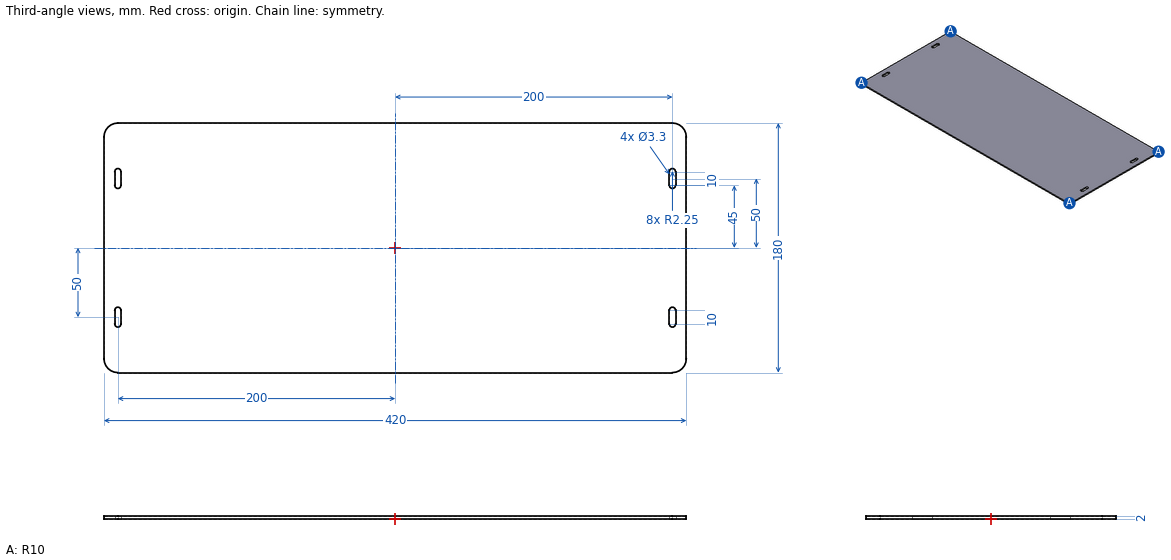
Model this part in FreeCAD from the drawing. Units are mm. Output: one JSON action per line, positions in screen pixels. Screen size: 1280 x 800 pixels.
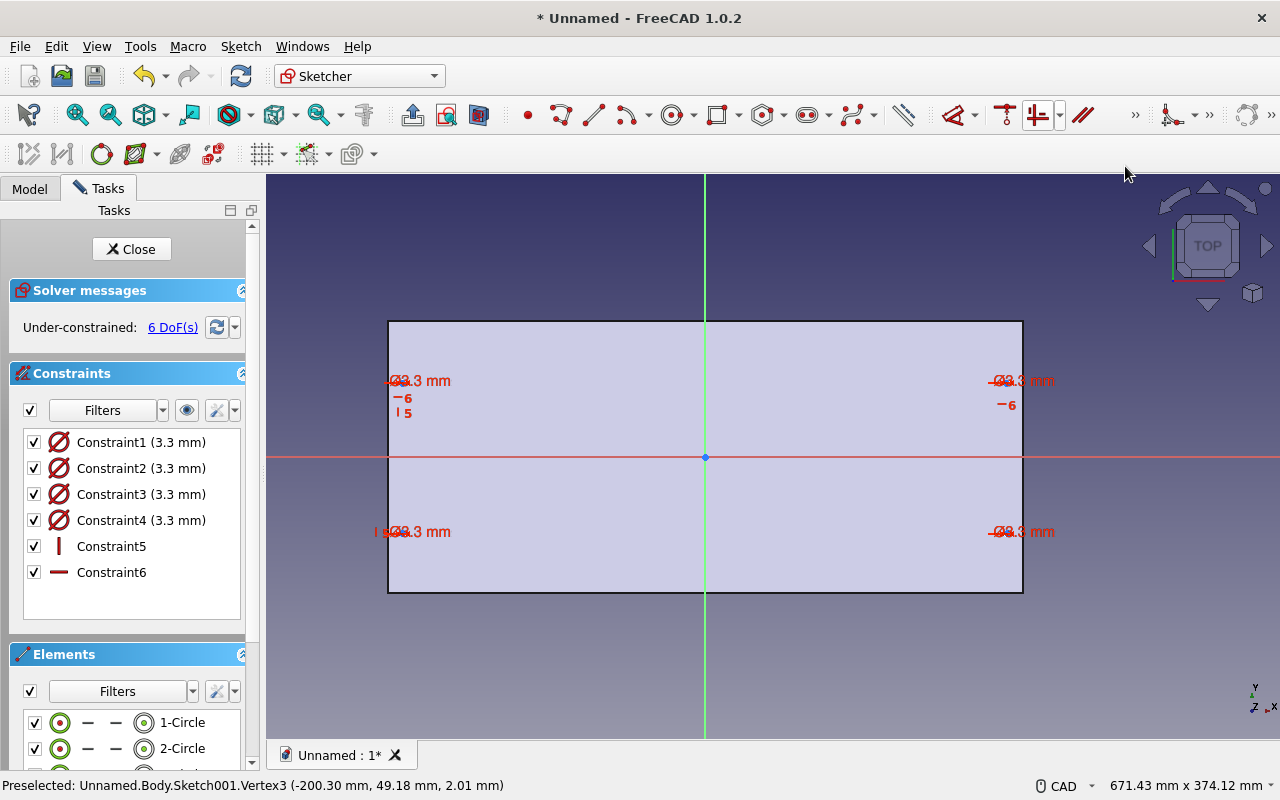
{"action": "left_click", "coordinate": [1007, 383]}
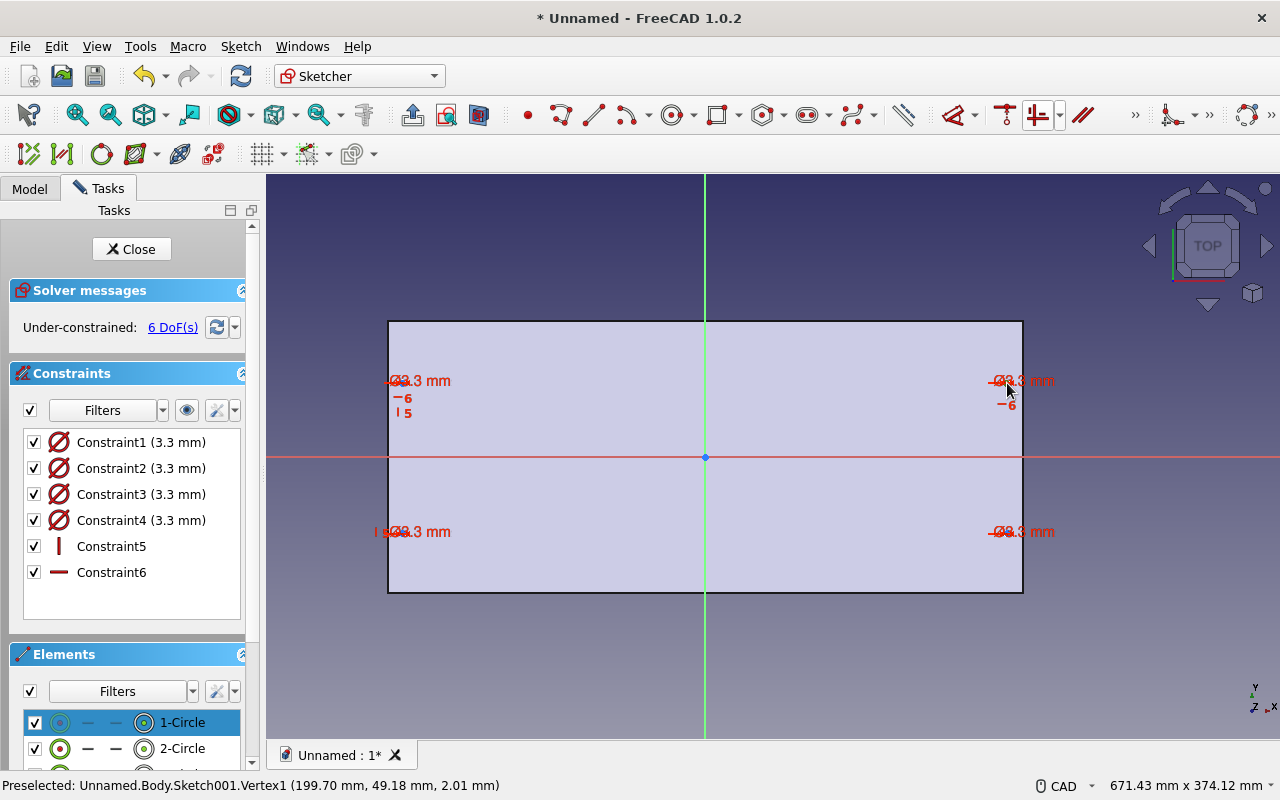
{"action": "left_click", "coordinate": [1007, 534]}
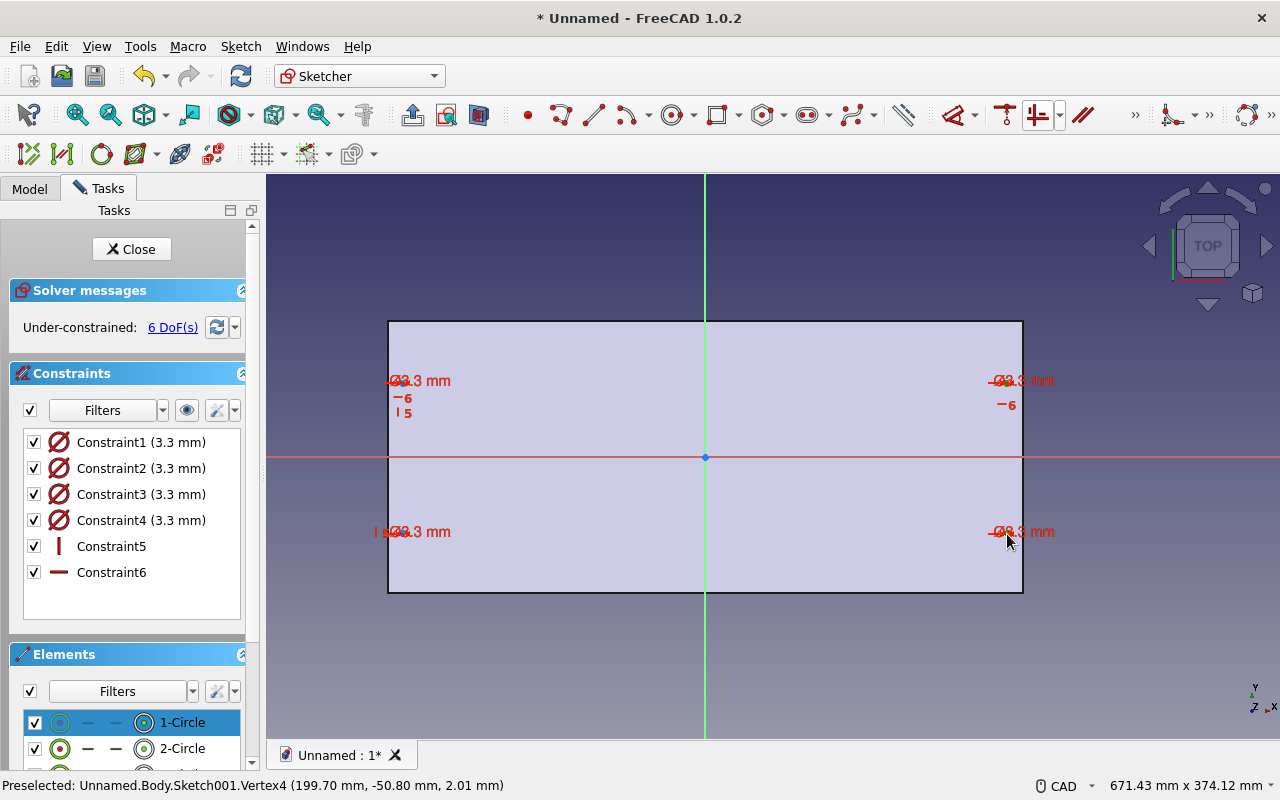
{"action": "key", "text": "v"}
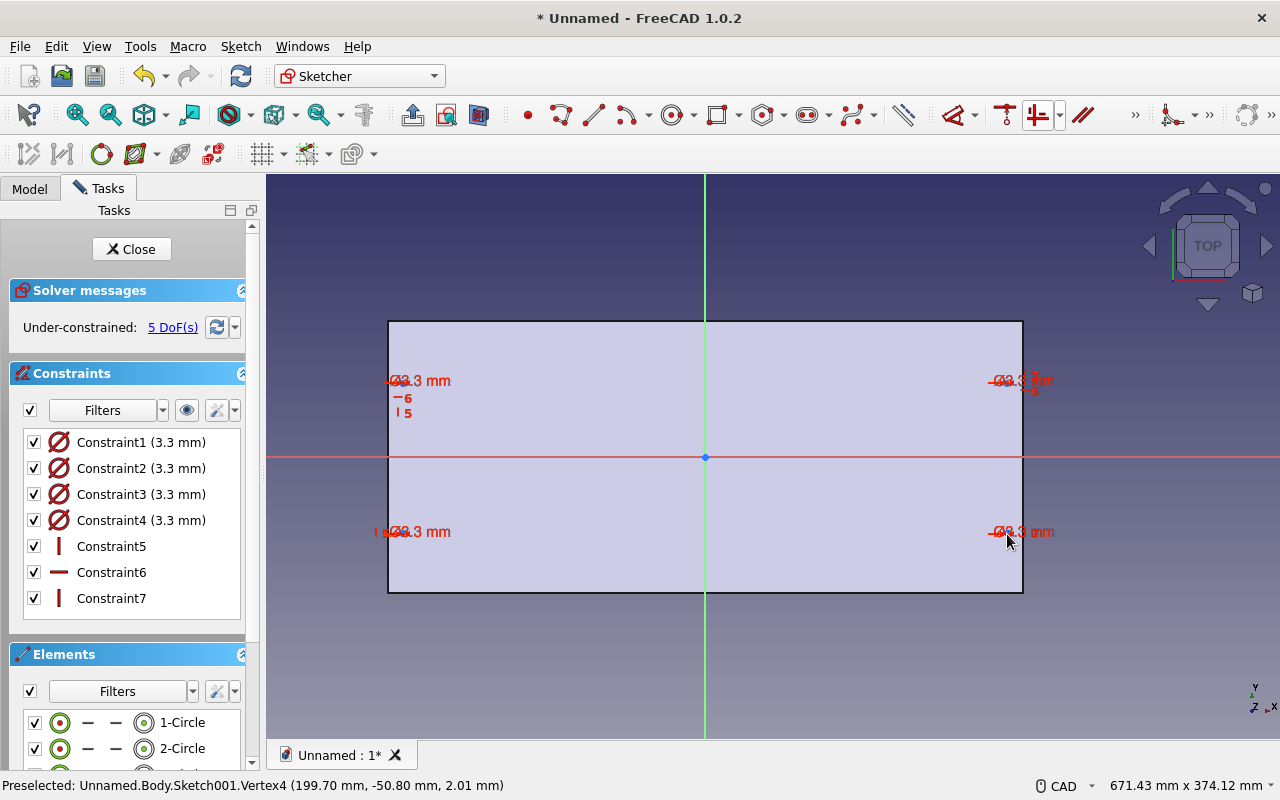
{"action": "left_click", "coordinate": [403, 534]}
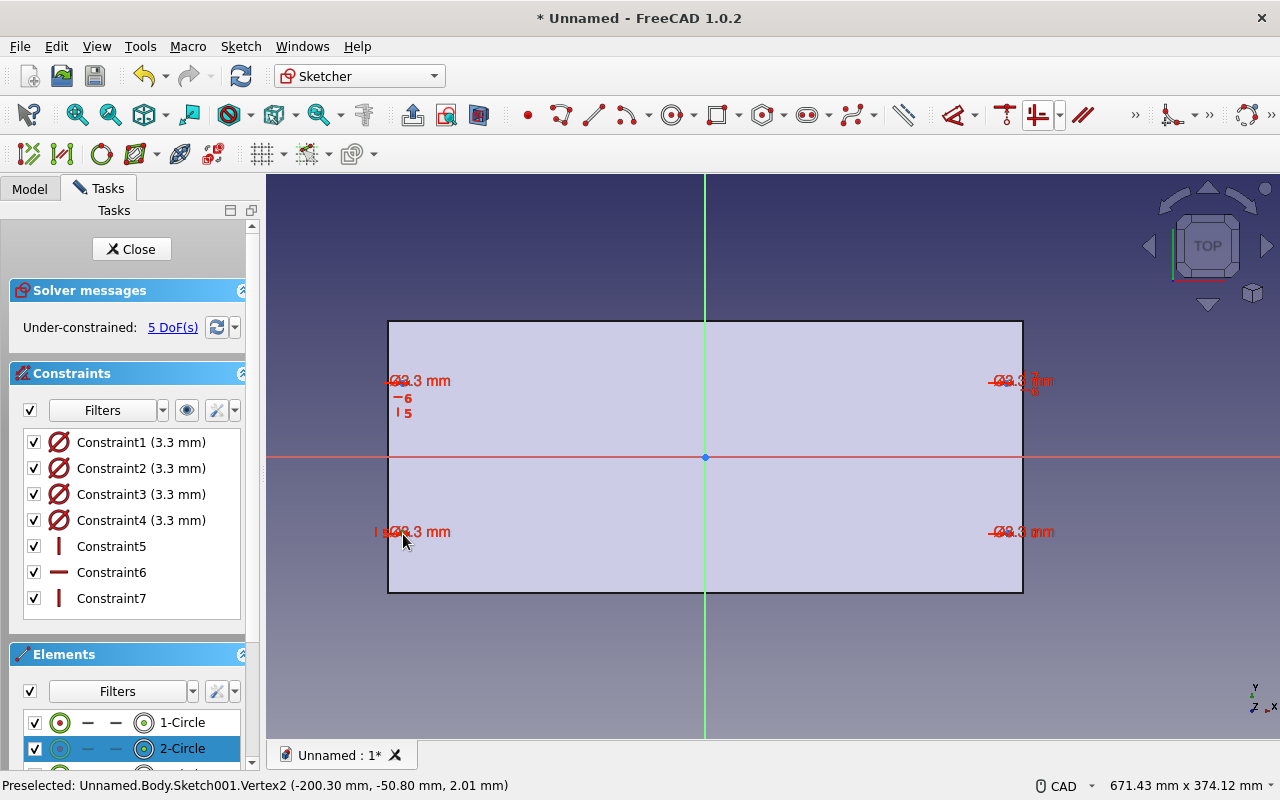
{"action": "left_click", "coordinate": [1007, 534]}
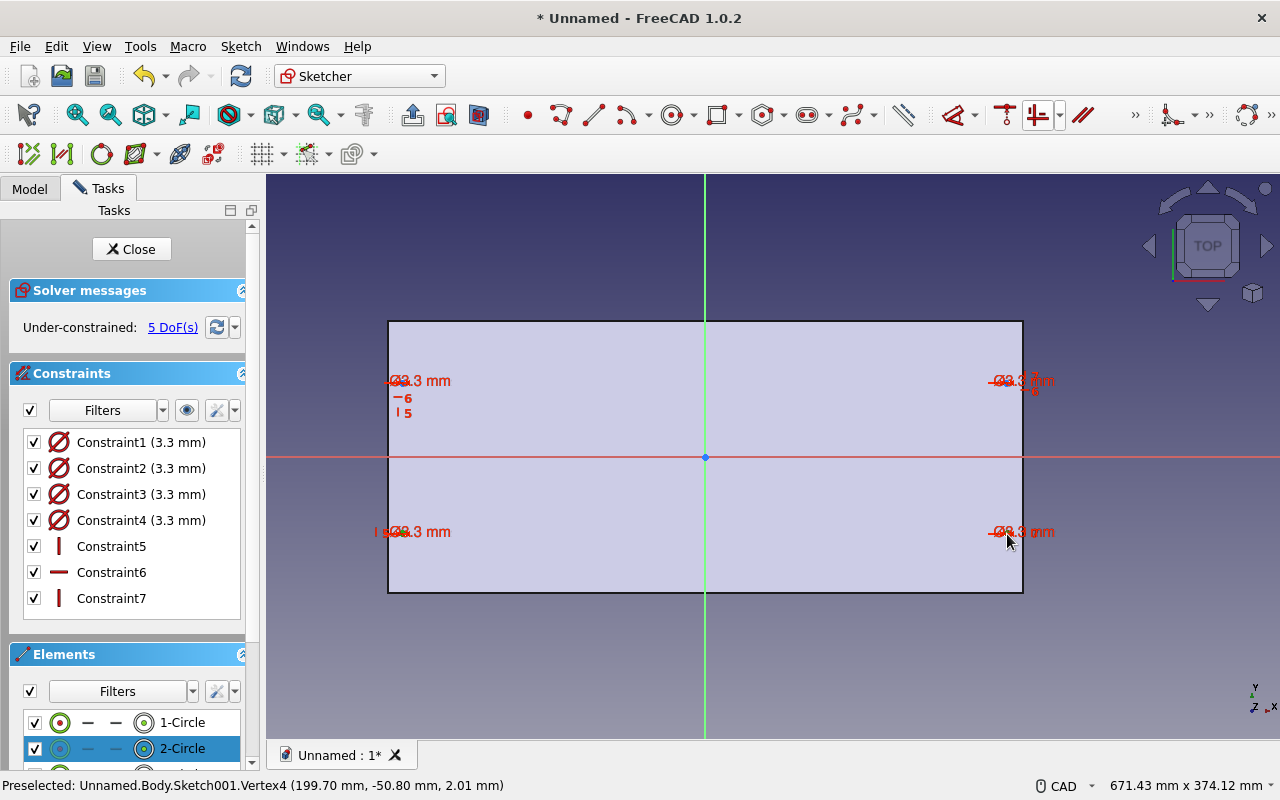
{"action": "key", "text": "h"}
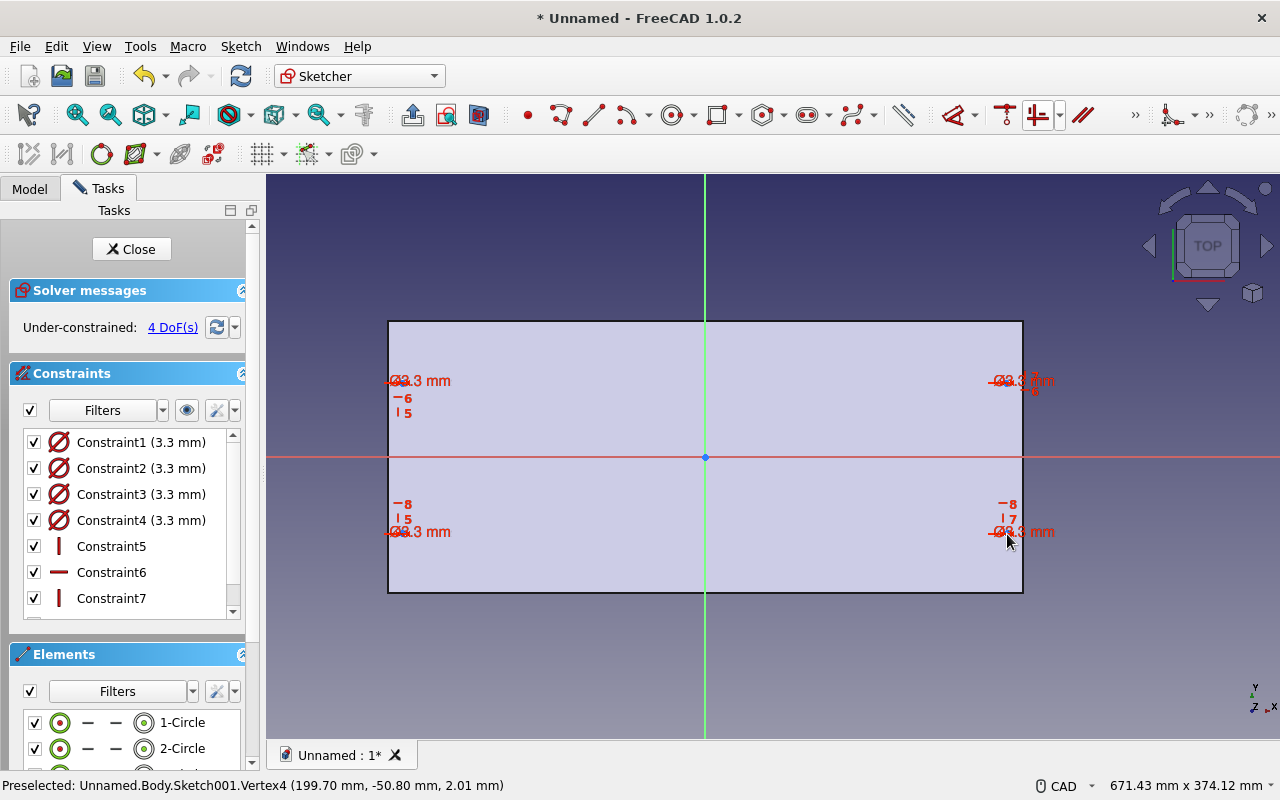
{"action": "key", "text": "d"}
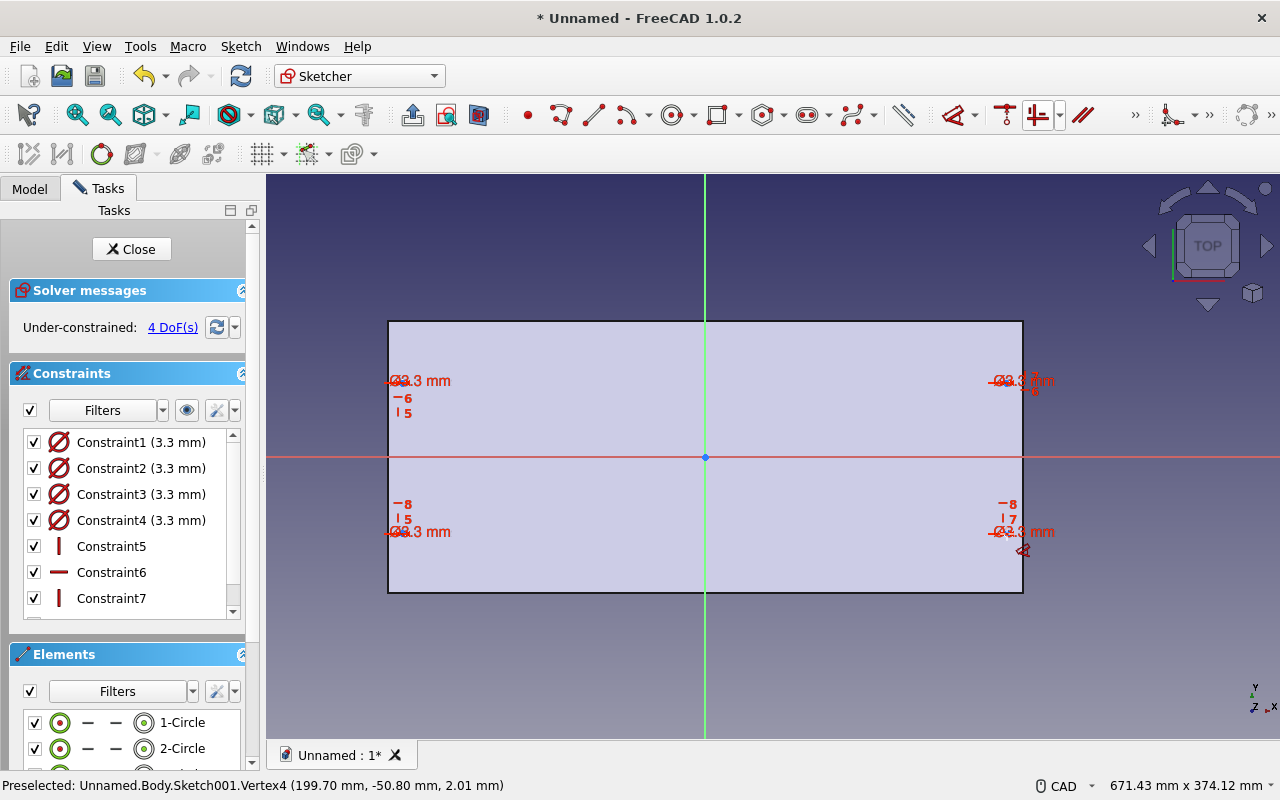
{"action": "left_click", "coordinate": [1007, 383]}
{"action": "left_click", "coordinate": [1041, 420]}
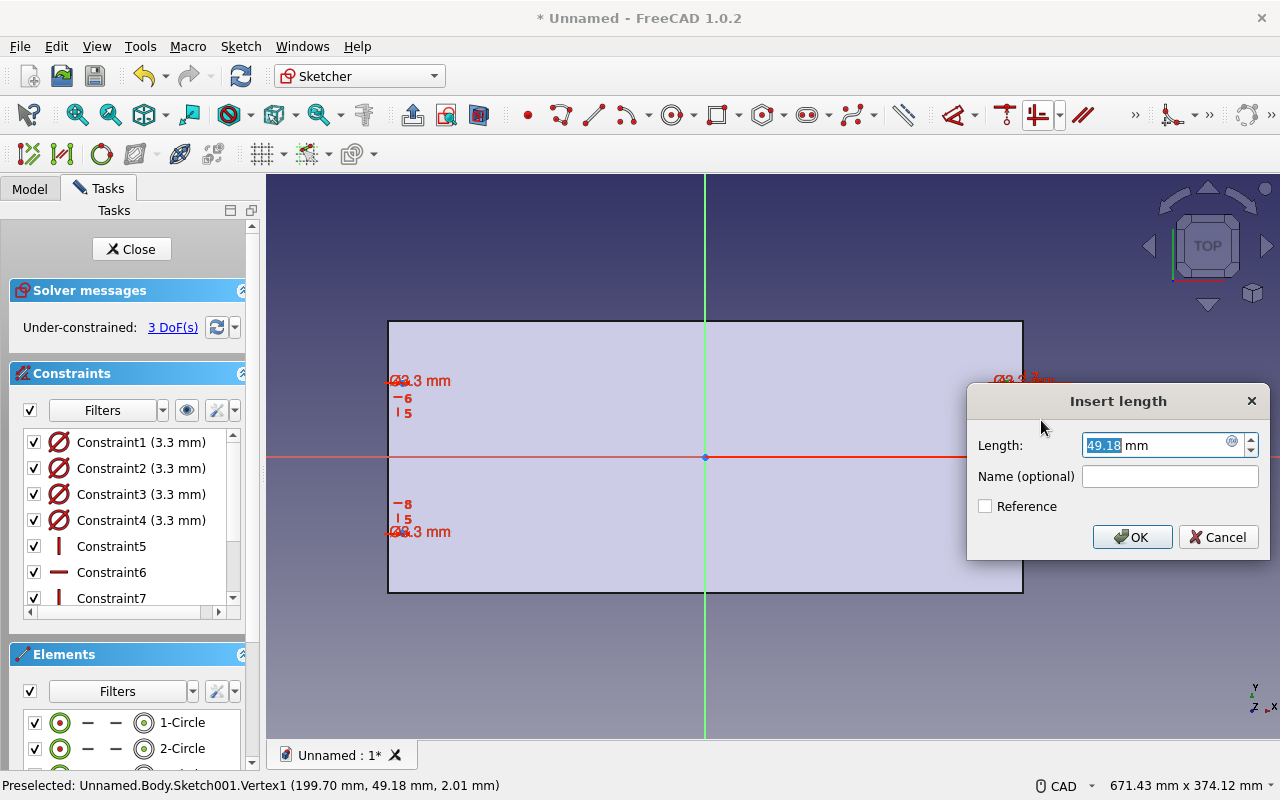
{"action": "type", "text": "50"}
{"action": "key", "text": "Return"}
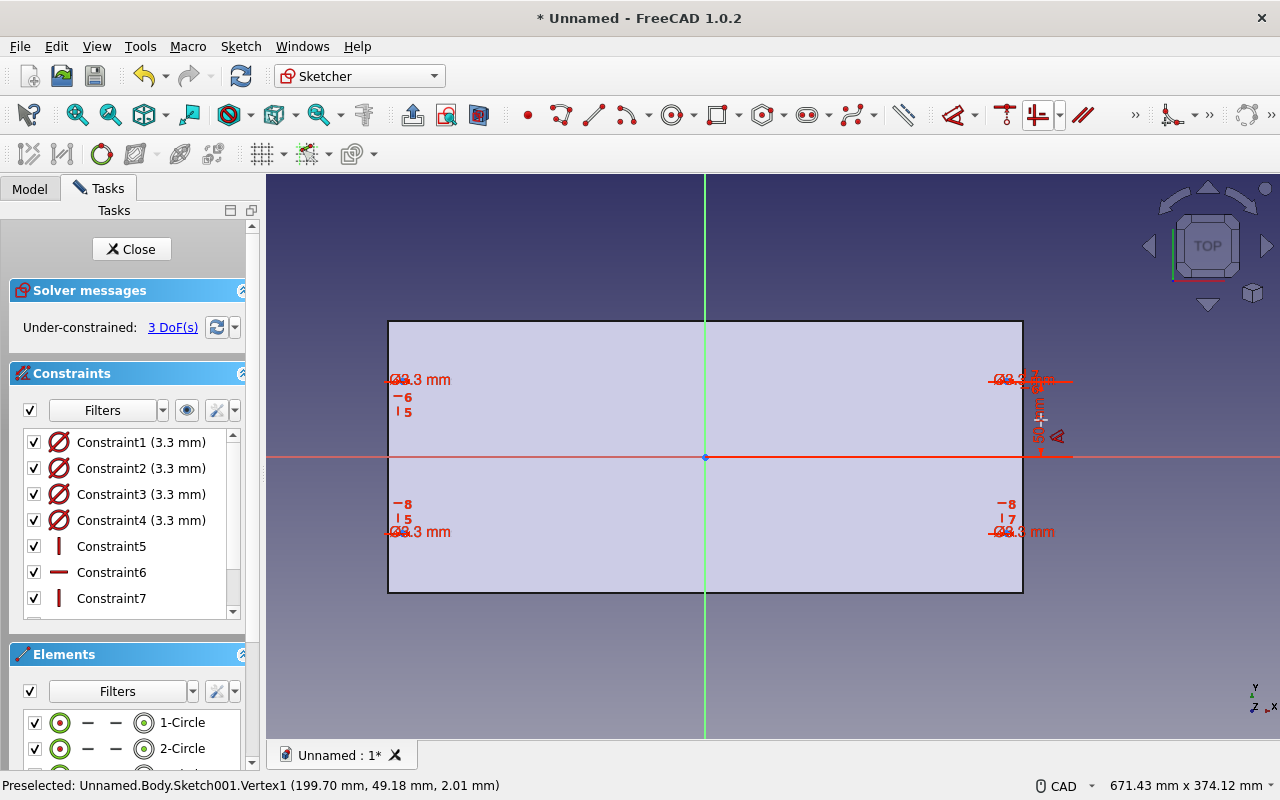
{"action": "left_click", "coordinate": [403, 534]}
{"action": "left_click", "coordinate": [369, 496]}